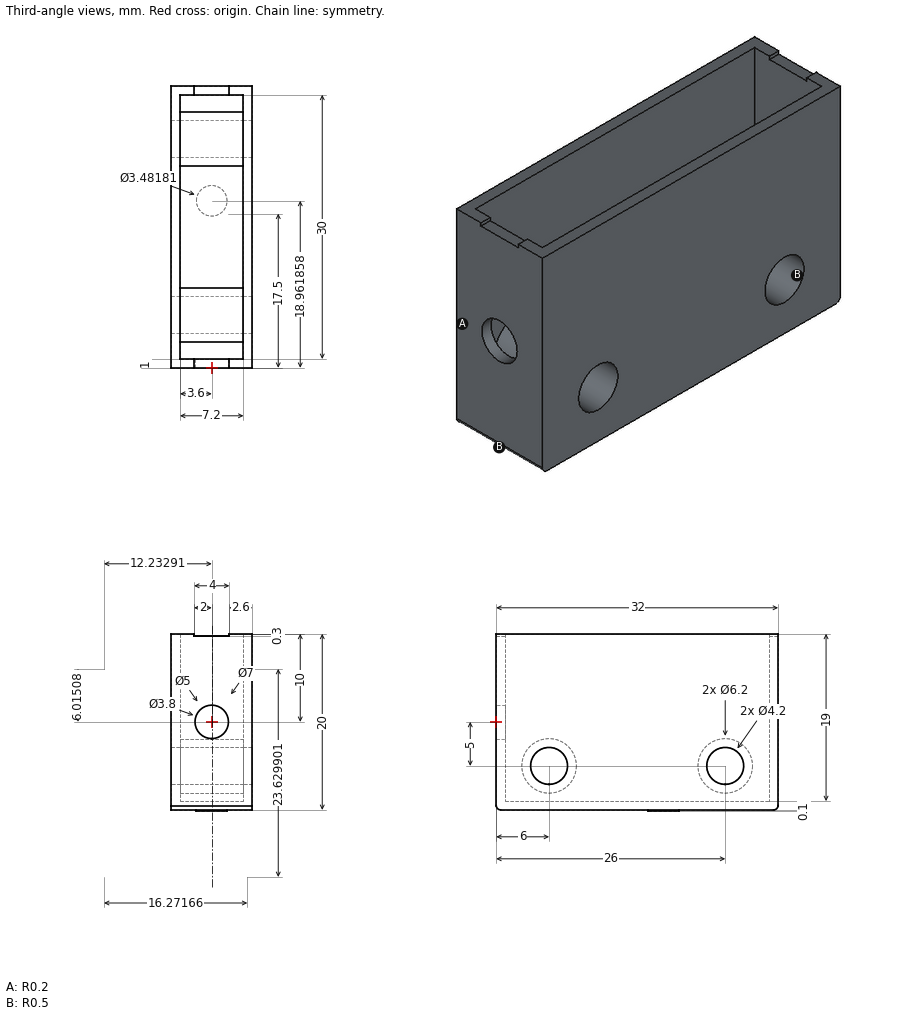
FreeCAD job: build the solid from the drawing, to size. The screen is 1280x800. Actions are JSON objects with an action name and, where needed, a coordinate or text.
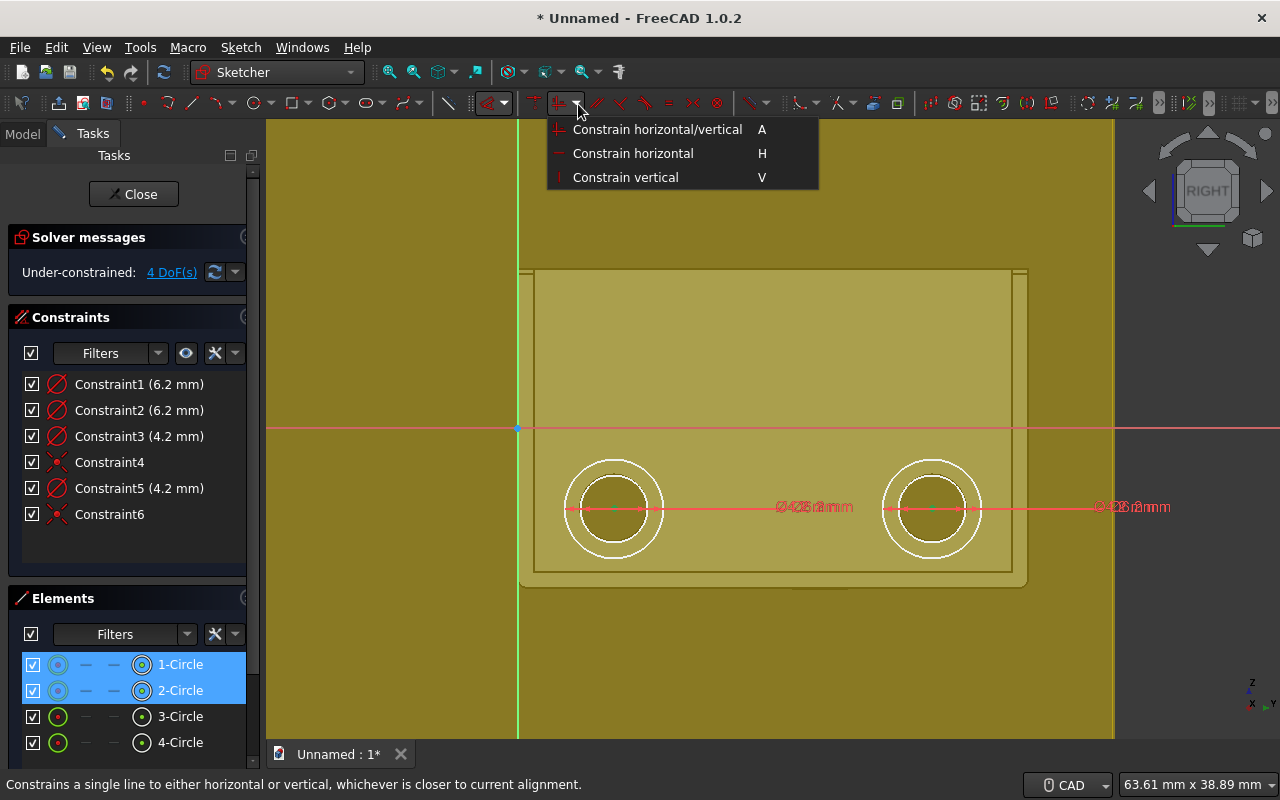
{"action": "left_click", "coordinate": [683, 153]}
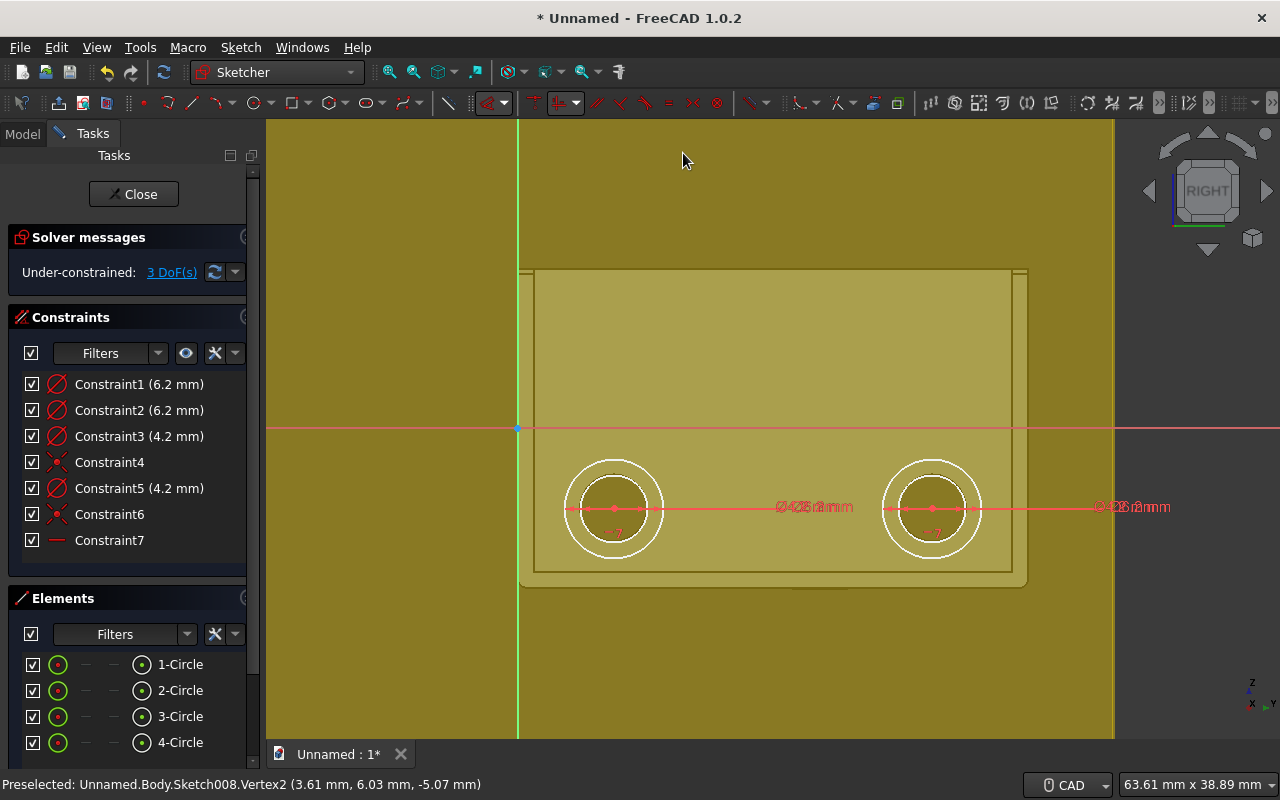
{"action": "left_click", "coordinate": [932, 509]}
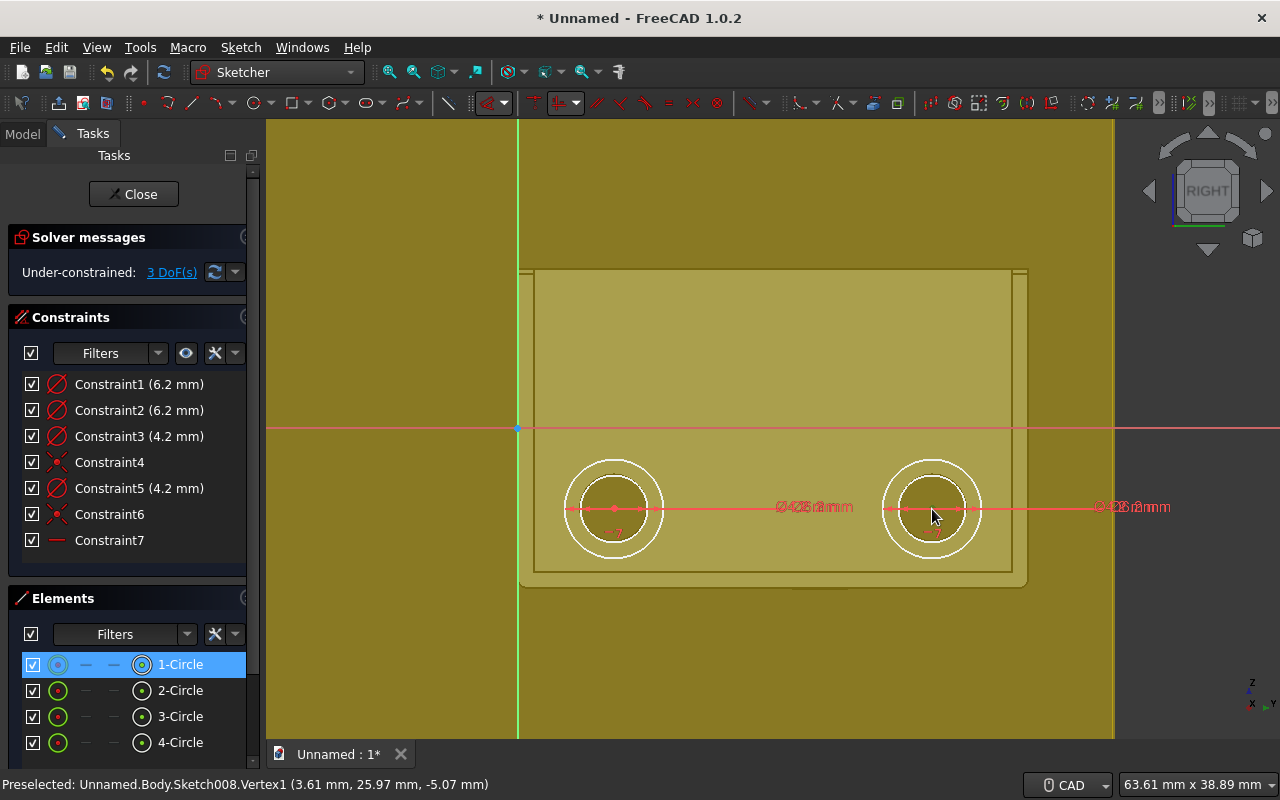
{"action": "key", "text": "i"}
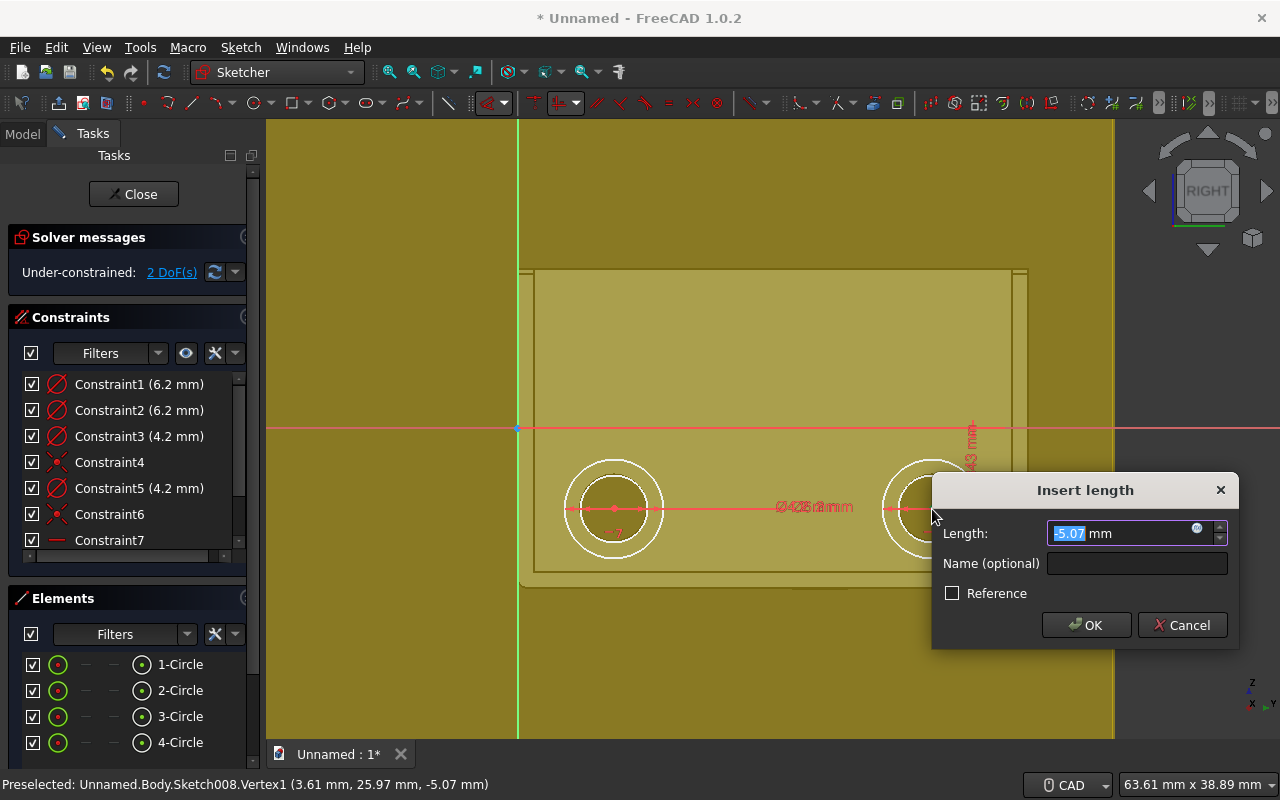
{"action": "type", "text": "-5"}
{"action": "key", "text": "Return"}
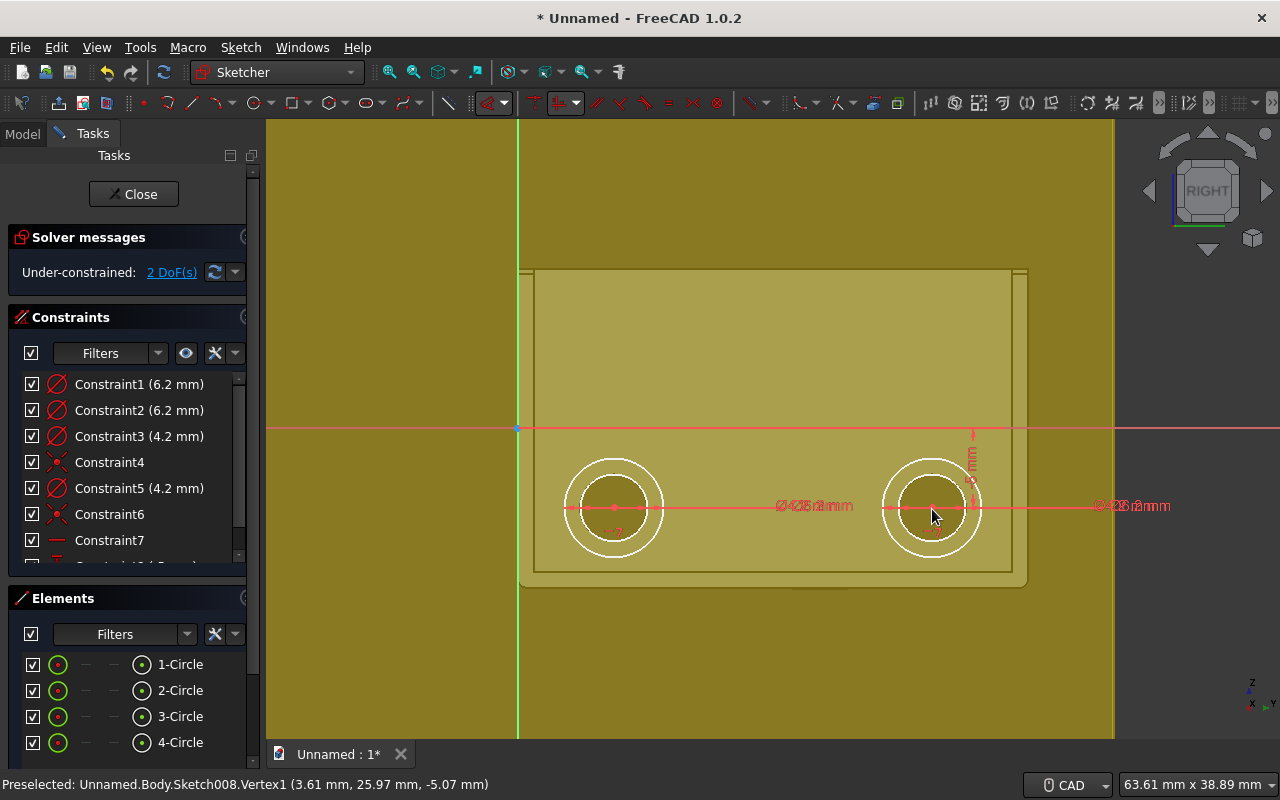
{"action": "left_click", "coordinate": [614, 508]}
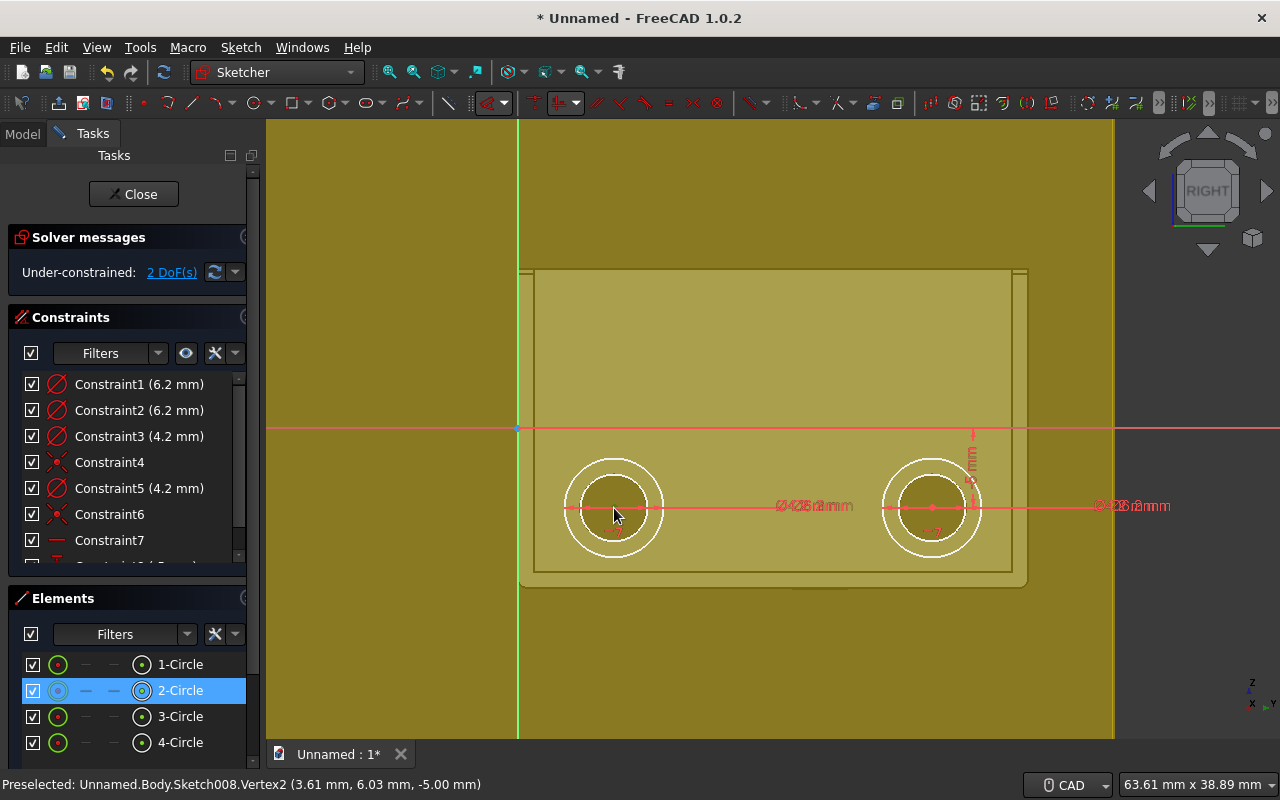
{"action": "left_click", "coordinate": [506, 104]}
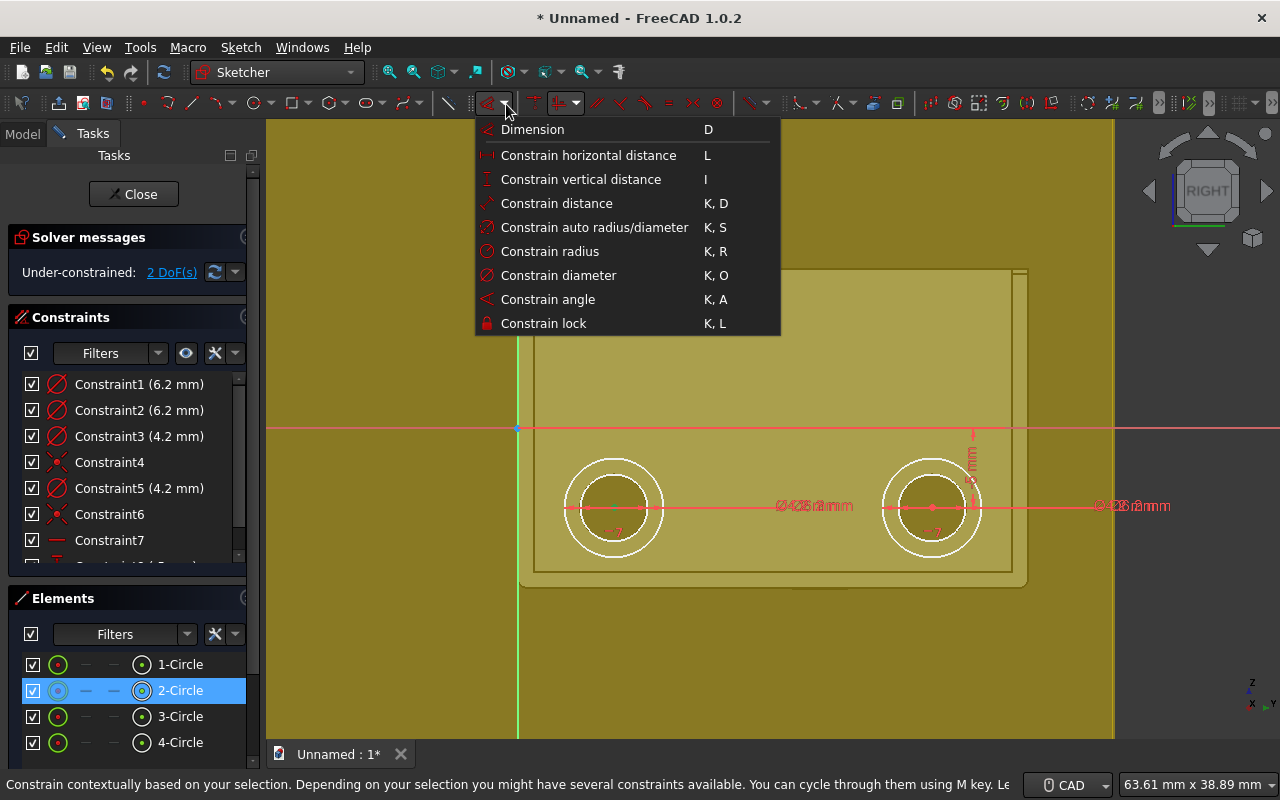
{"action": "left_click", "coordinate": [628, 155]}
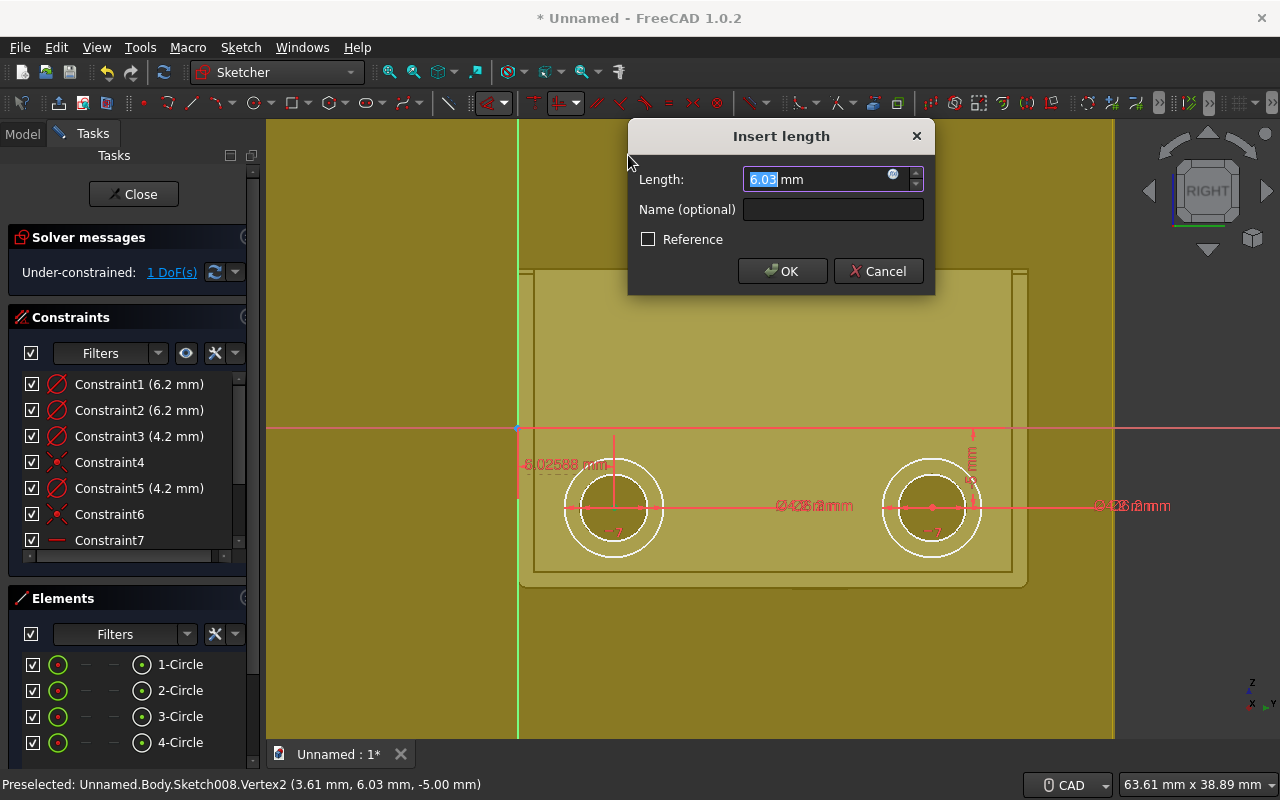
{"action": "type", "text": "6"}
{"action": "key", "text": "Return"}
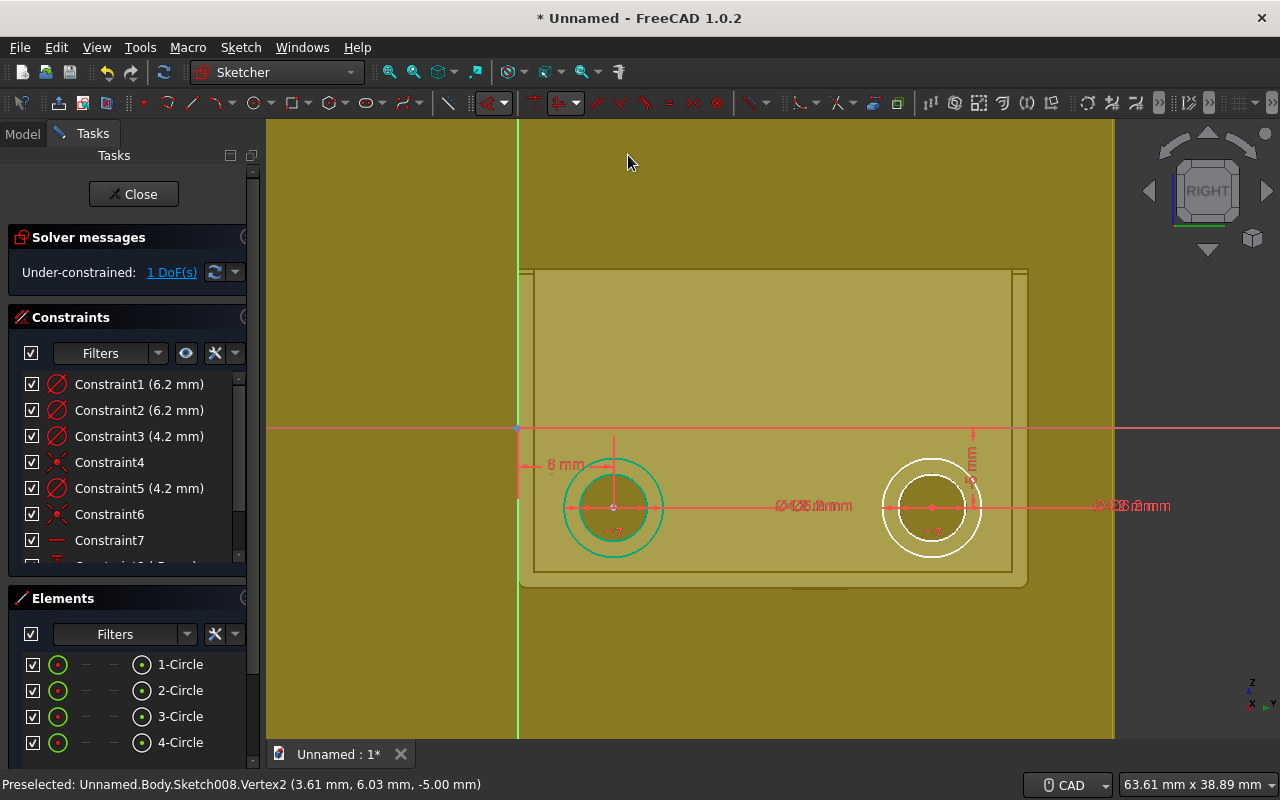
{"action": "left_click", "coordinate": [932, 508]}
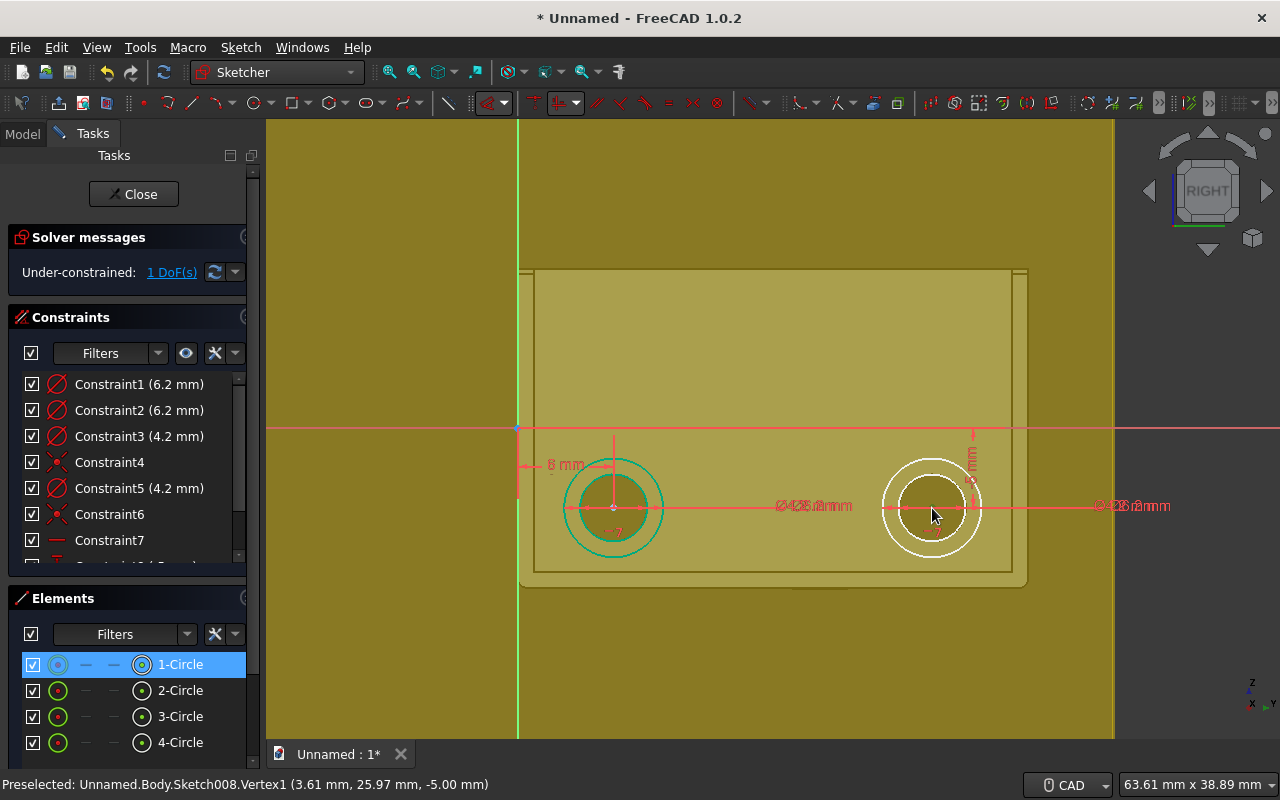
{"action": "left_click", "coordinate": [506, 104]}